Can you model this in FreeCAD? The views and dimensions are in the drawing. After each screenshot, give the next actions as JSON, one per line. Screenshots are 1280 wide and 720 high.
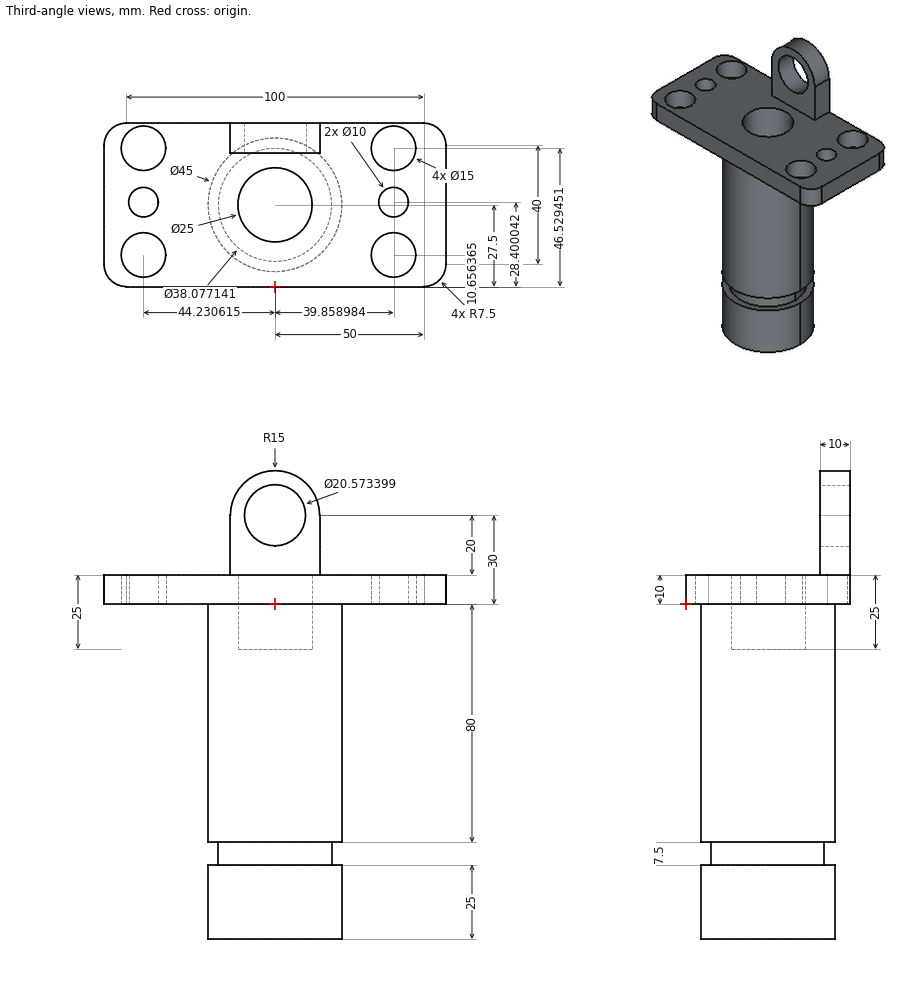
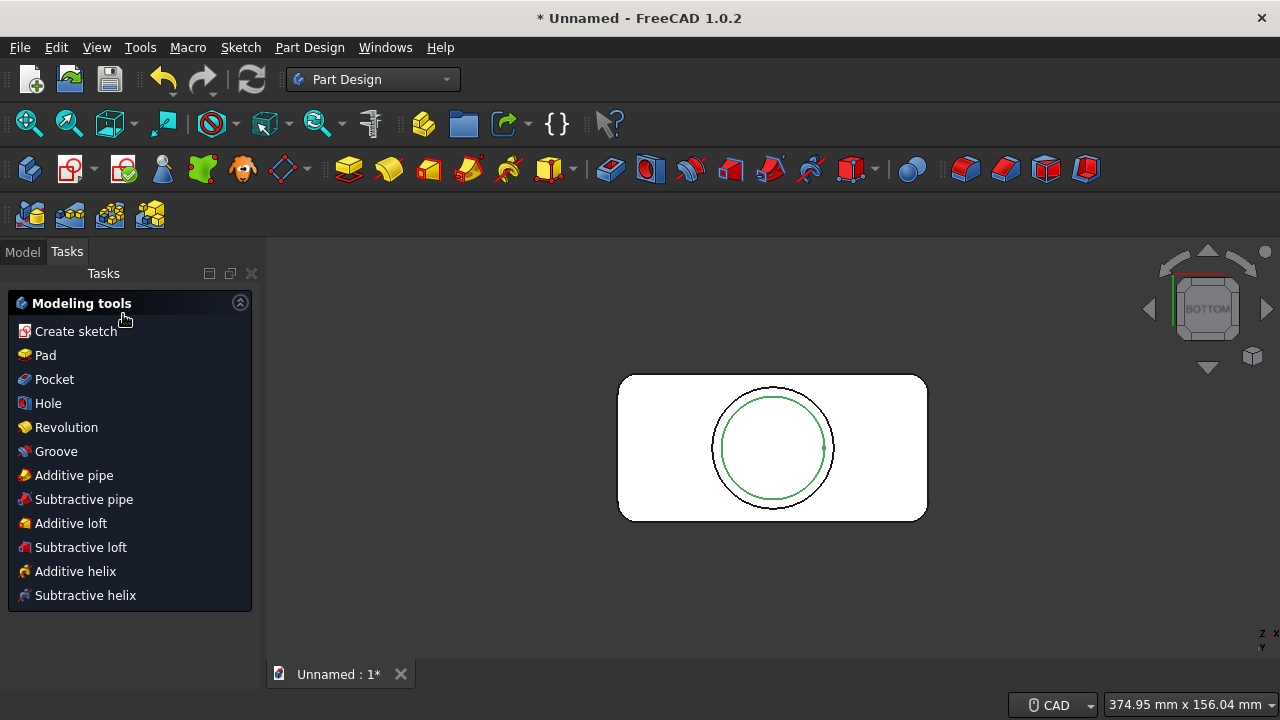
{"action": "left_click", "coordinate": [350, 170]}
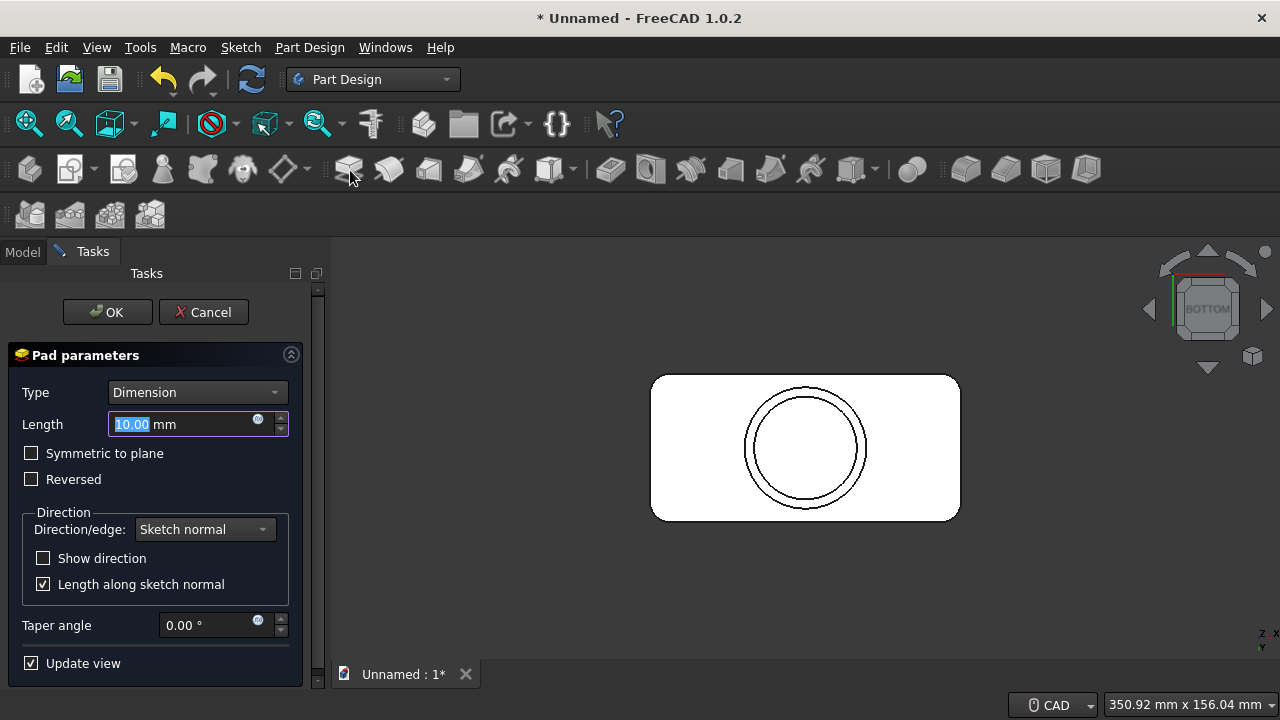
{"action": "type", "text": "7.5"}
{"action": "key", "text": "Tab"}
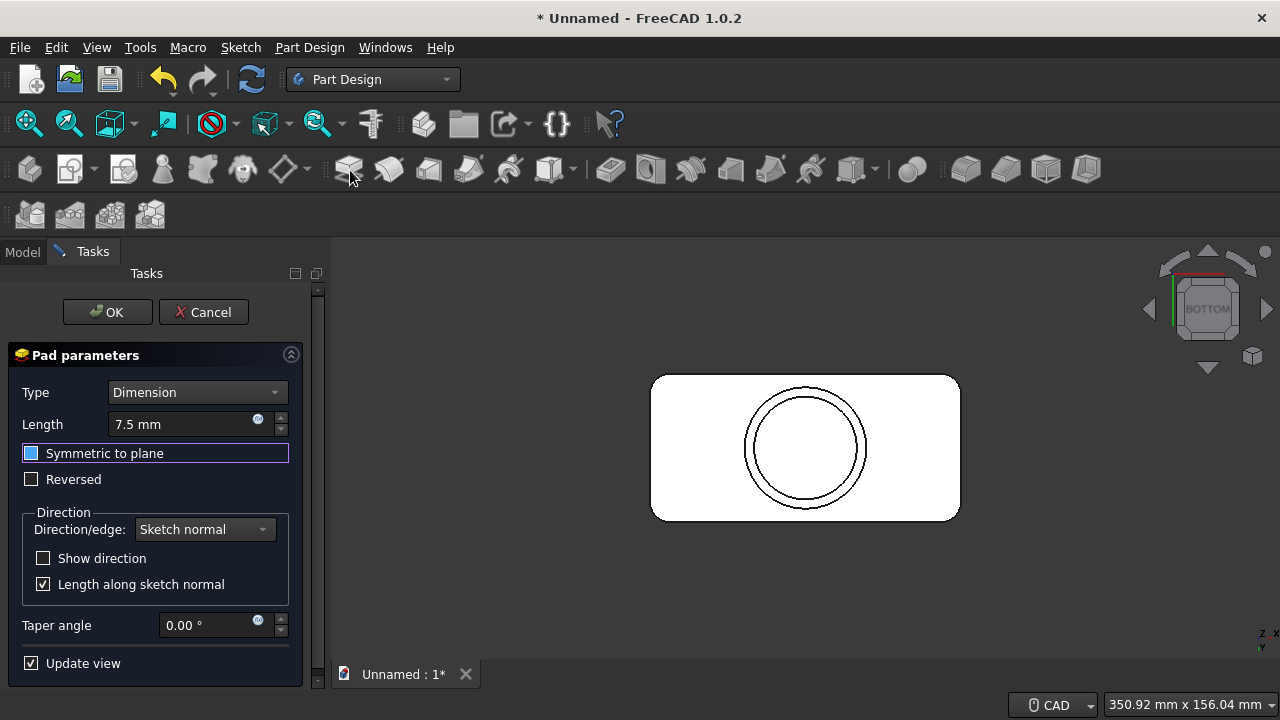
{"action": "left_click", "coordinate": [108, 312]}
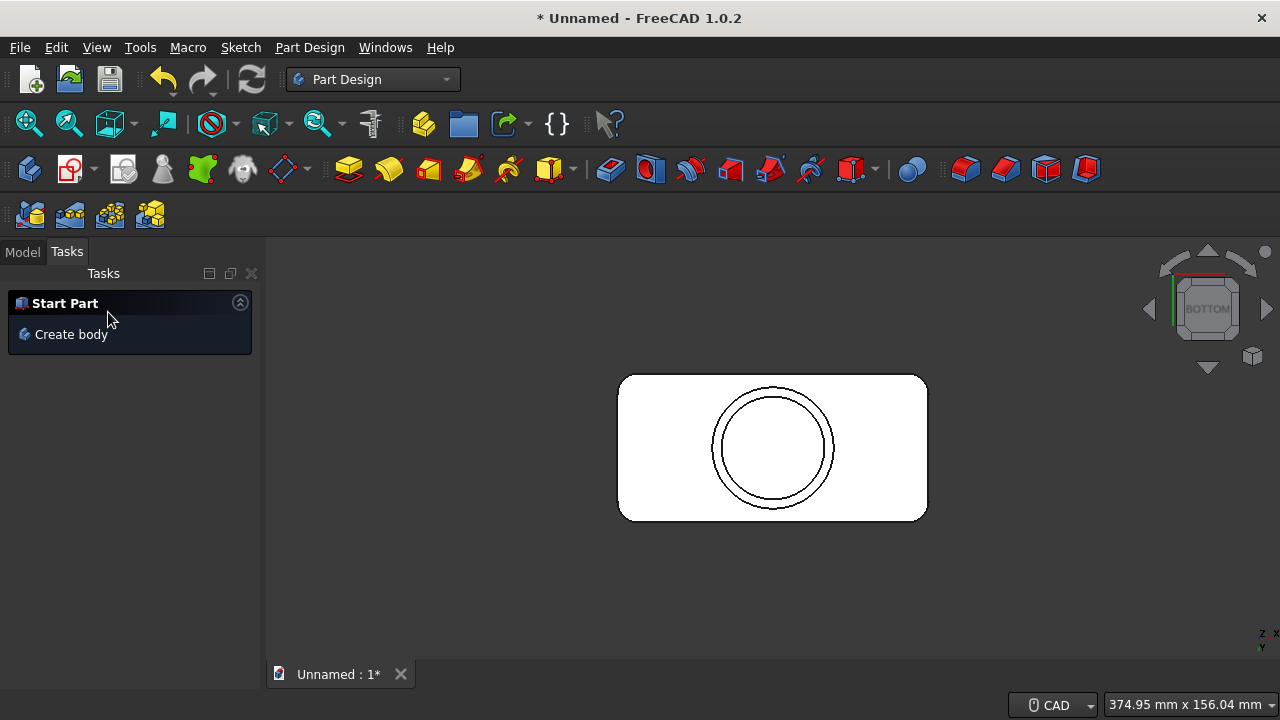
{"action": "key", "text": "v f"}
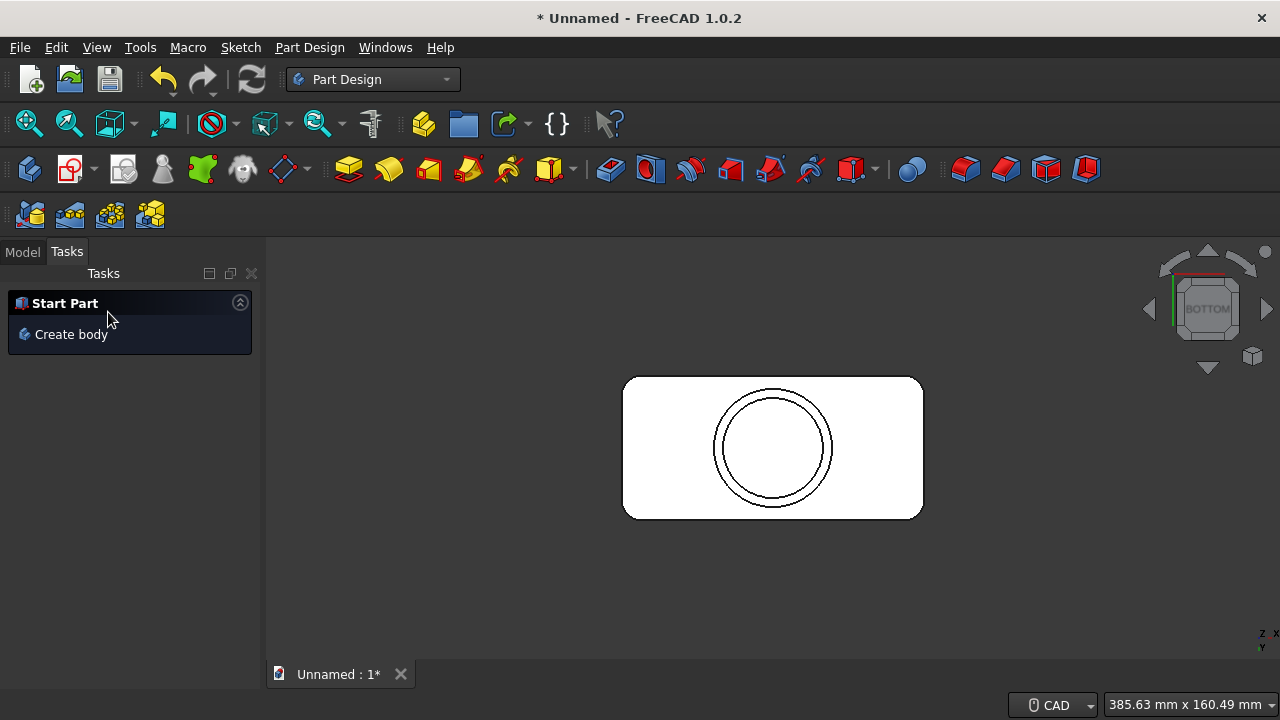
{"action": "left_click", "coordinate": [773, 447]}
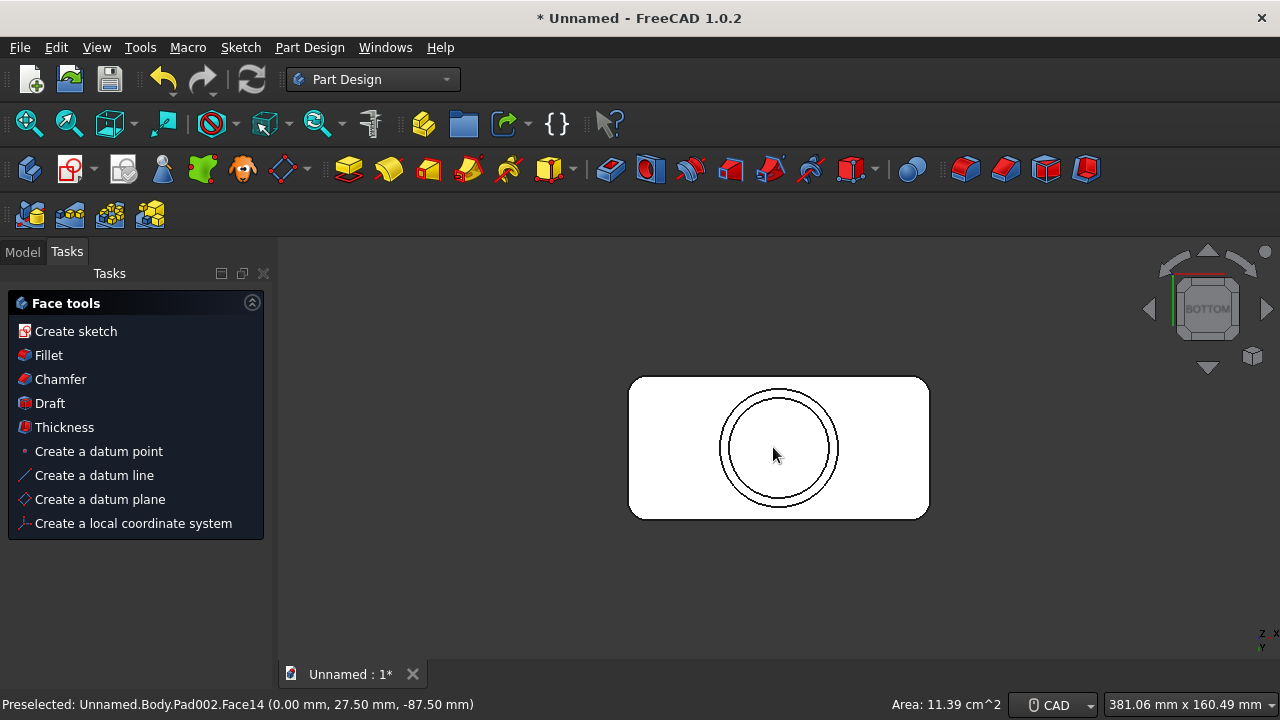
{"action": "left_click", "coordinate": [70, 170]}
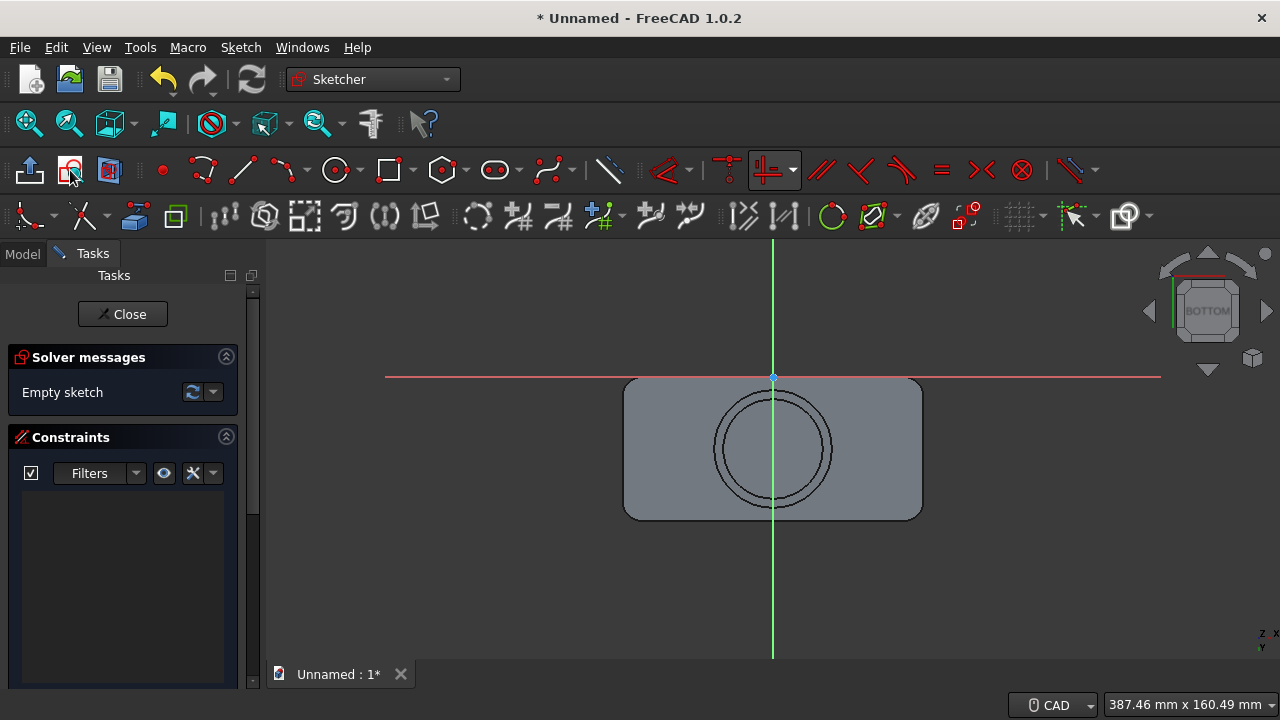
{"action": "scroll", "coordinate": [856, 434], "scroll_direction": "up", "scroll_amount": 3}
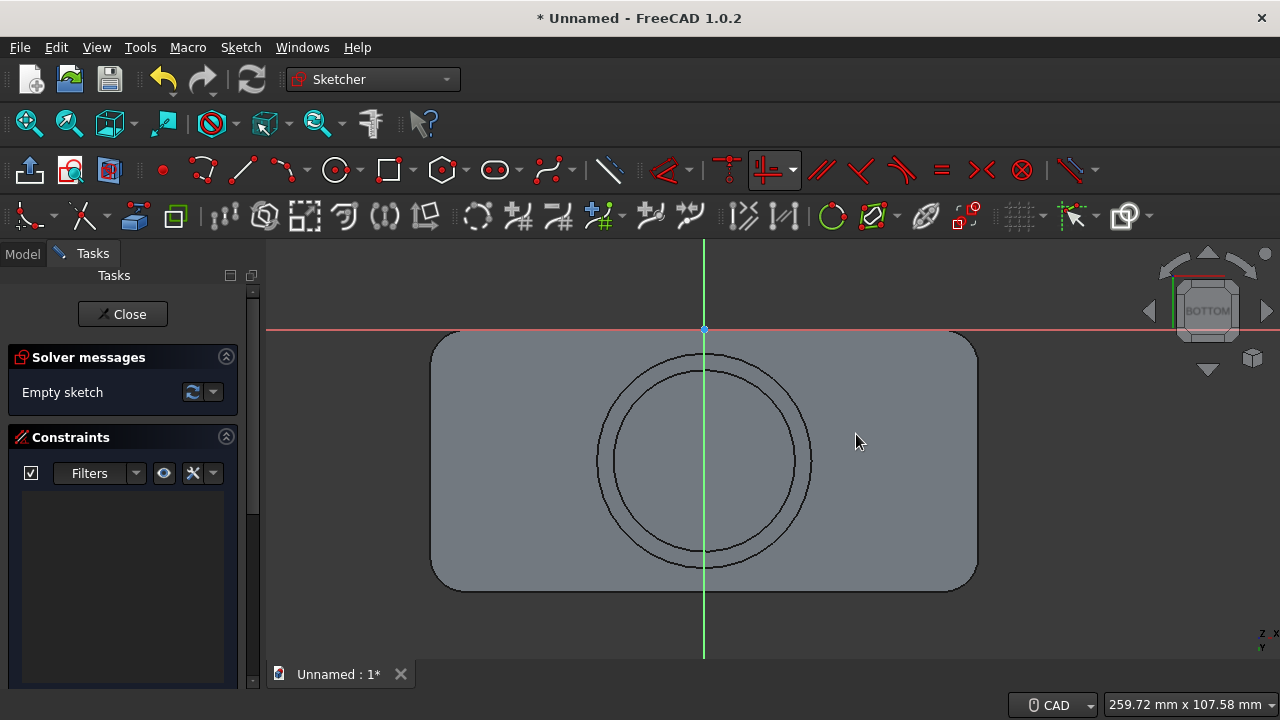
{"action": "left_click", "coordinate": [336, 170]}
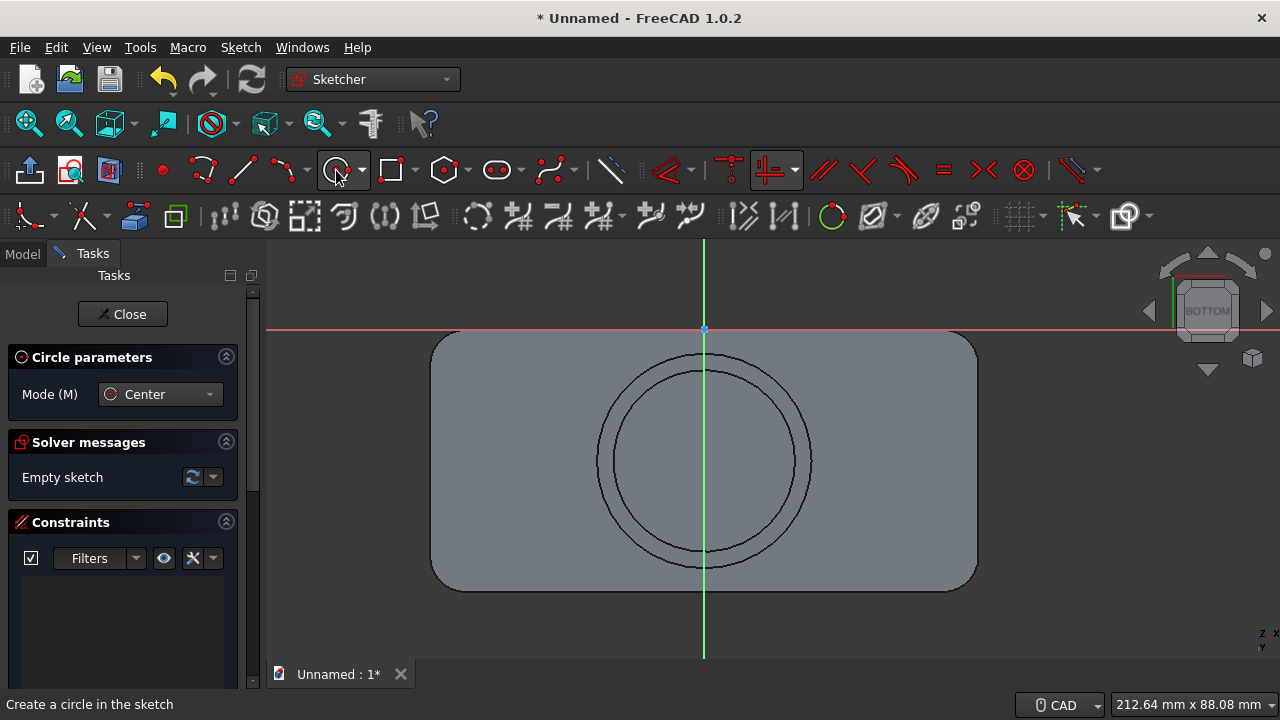
{"action": "left_click", "coordinate": [704, 461]}
{"action": "left_click", "coordinate": [780, 385]}
{"action": "key", "text": "Escape"}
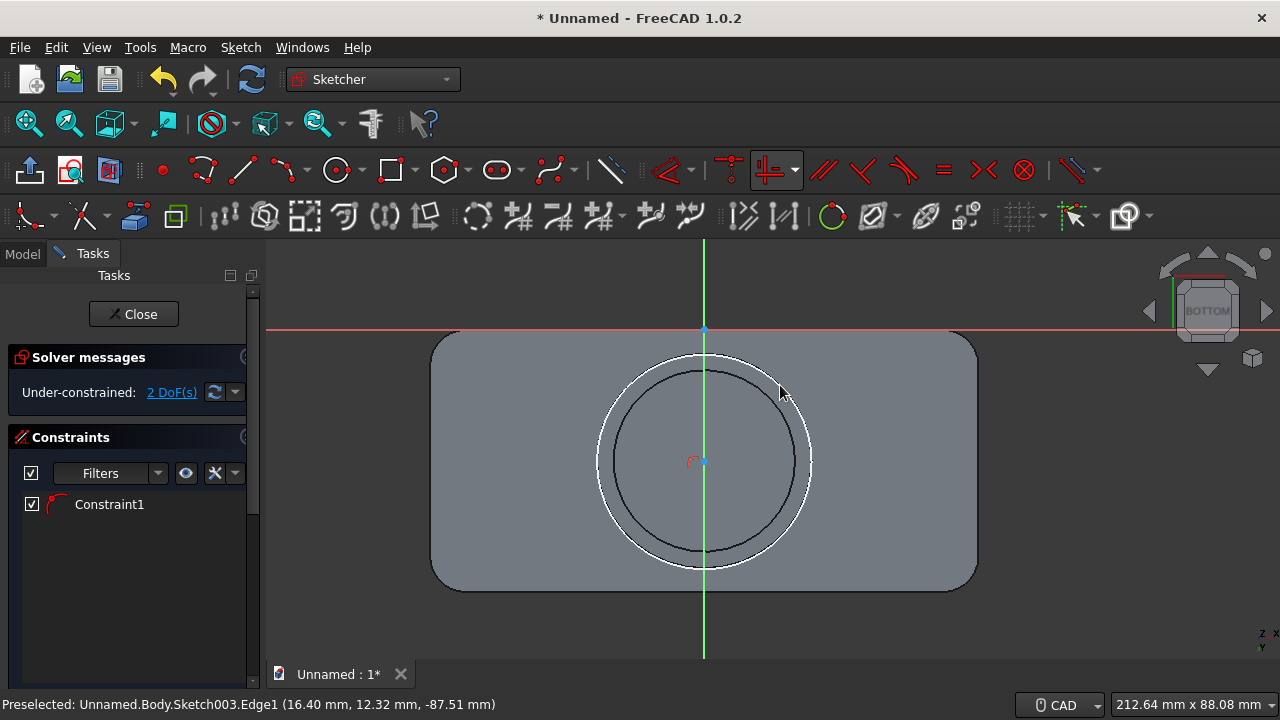
{"action": "key", "text": "d"}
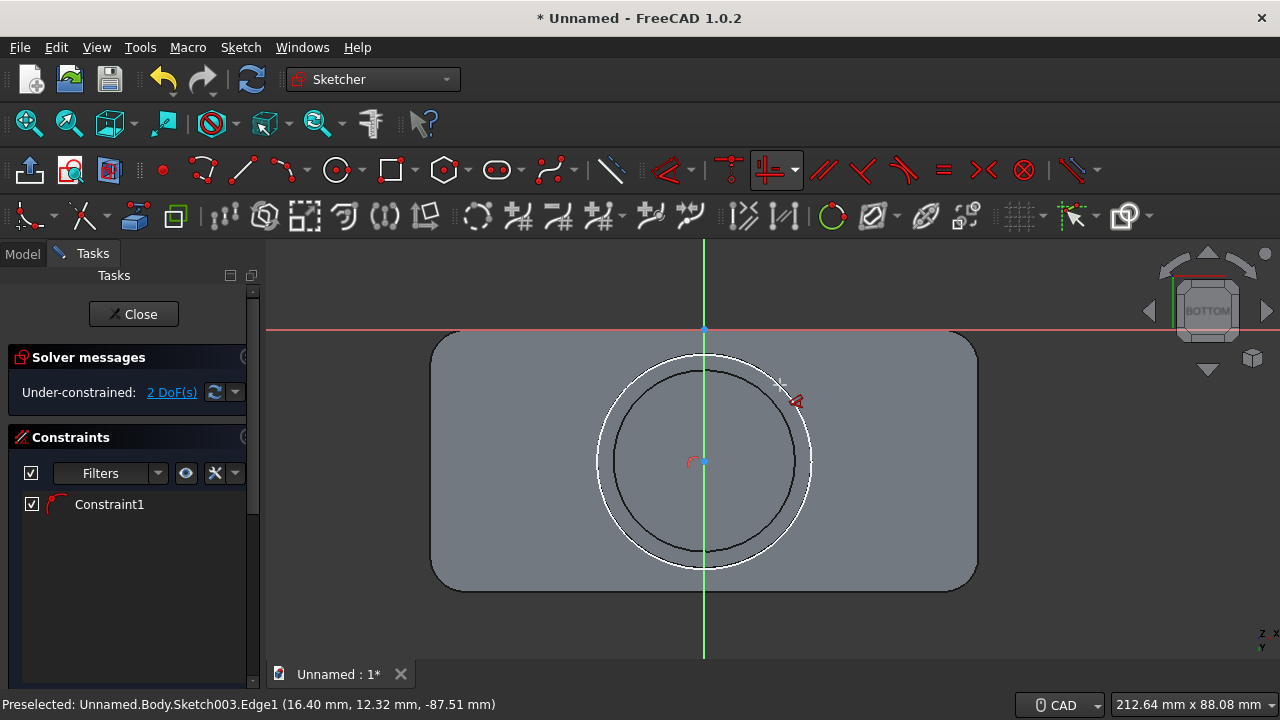
{"action": "left_click", "coordinate": [780, 386]}
{"action": "left_click", "coordinate": [803, 363]}